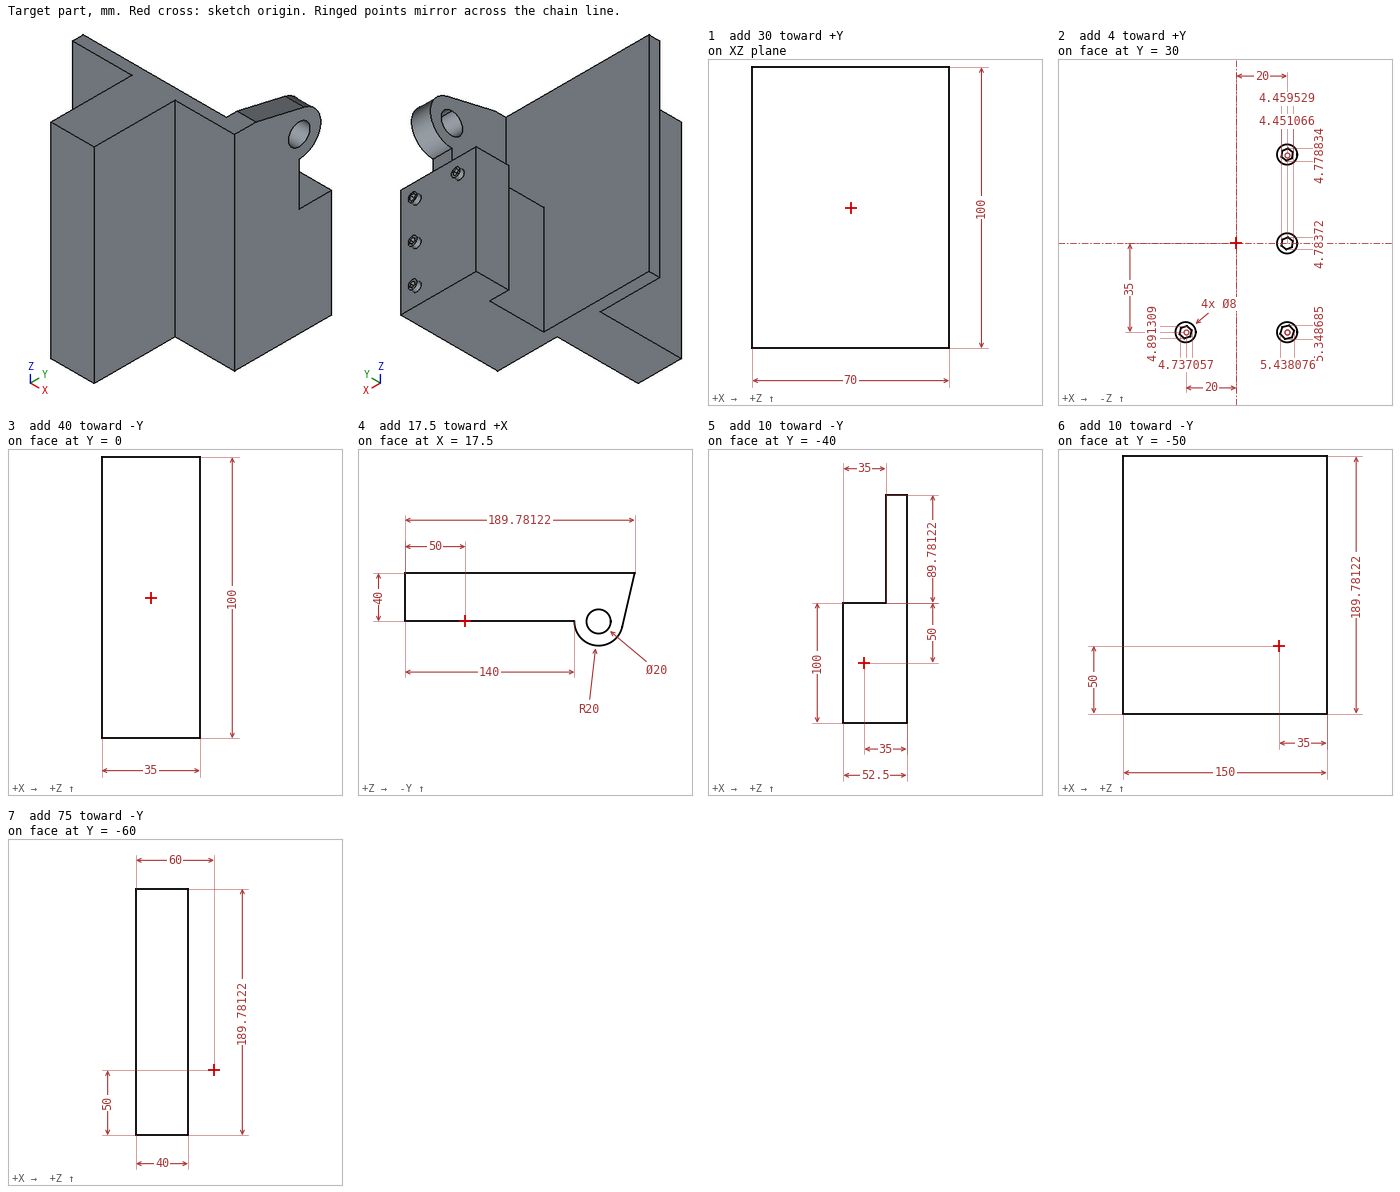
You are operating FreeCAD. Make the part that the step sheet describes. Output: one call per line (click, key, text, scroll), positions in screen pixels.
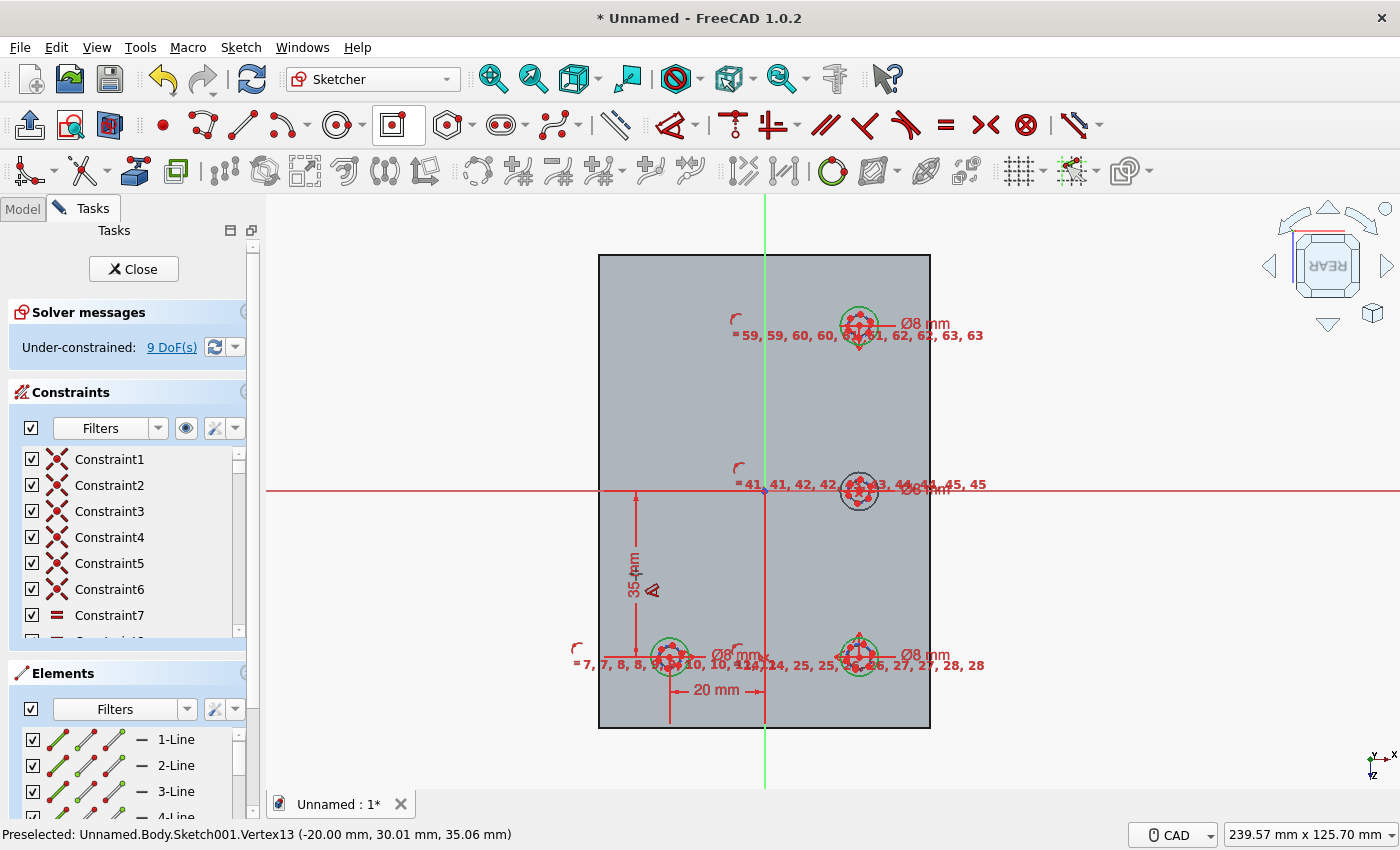
click(859, 491)
click(812, 525)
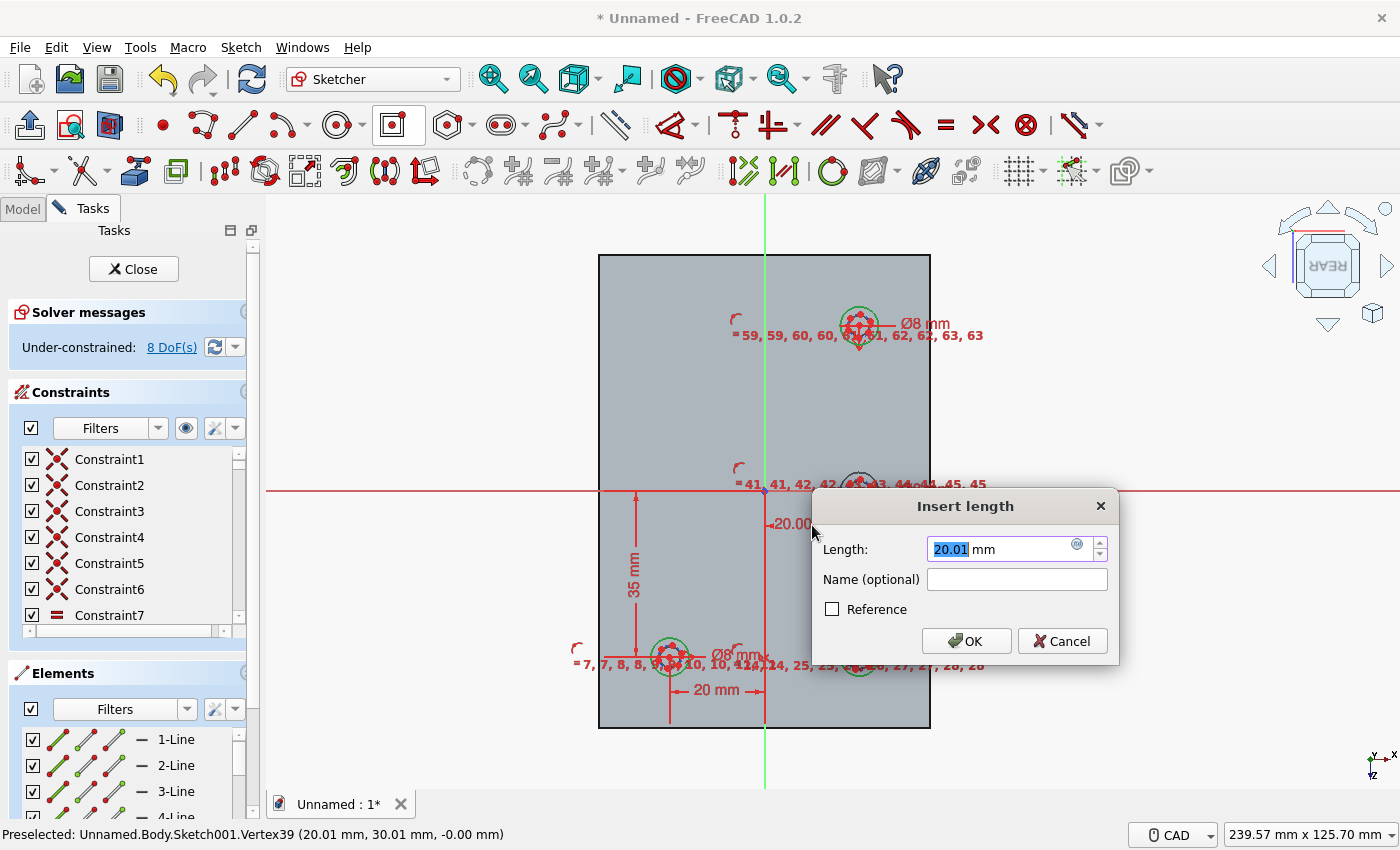
text(20)
key(Return)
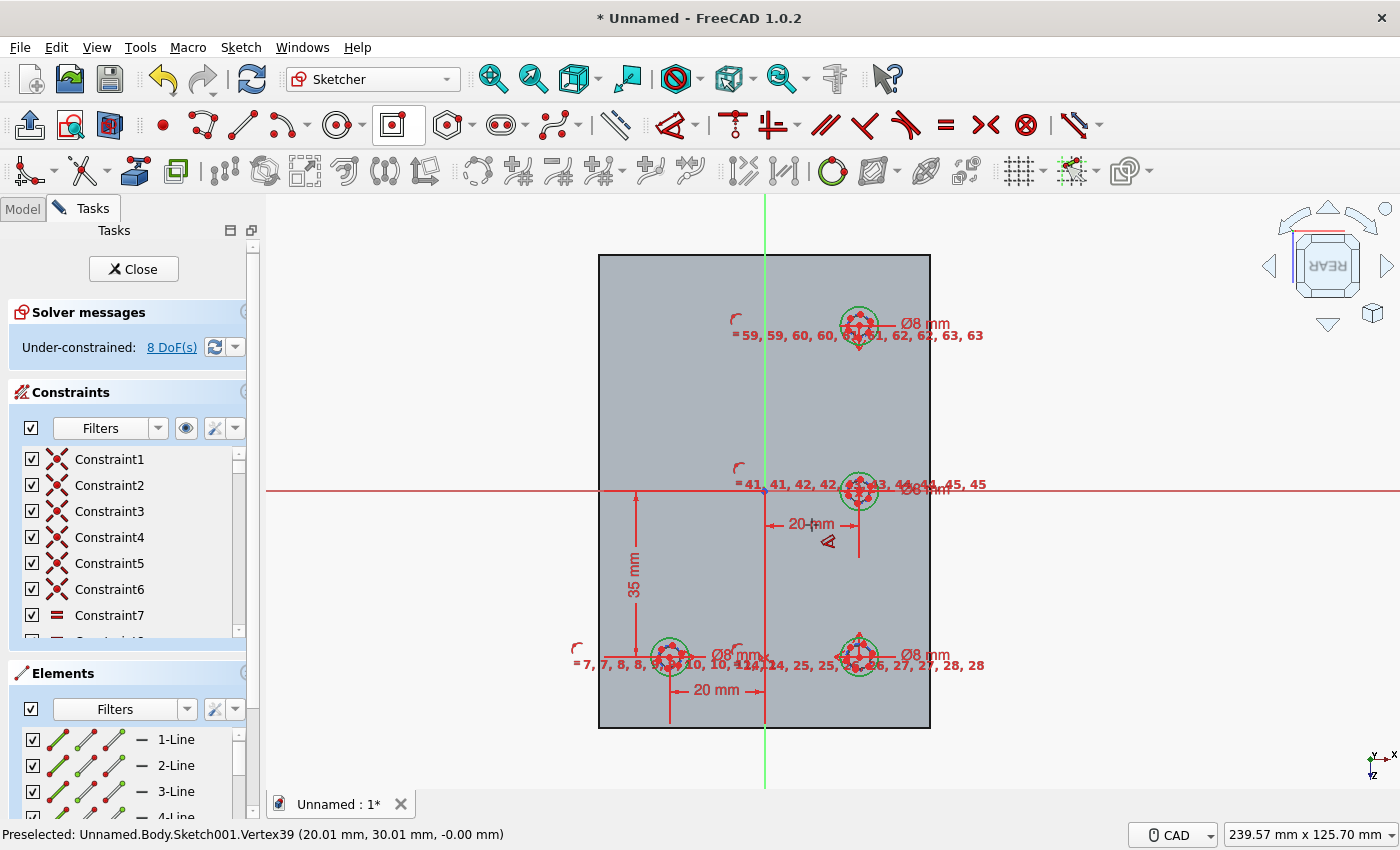
scroll(659, 660, up, 3)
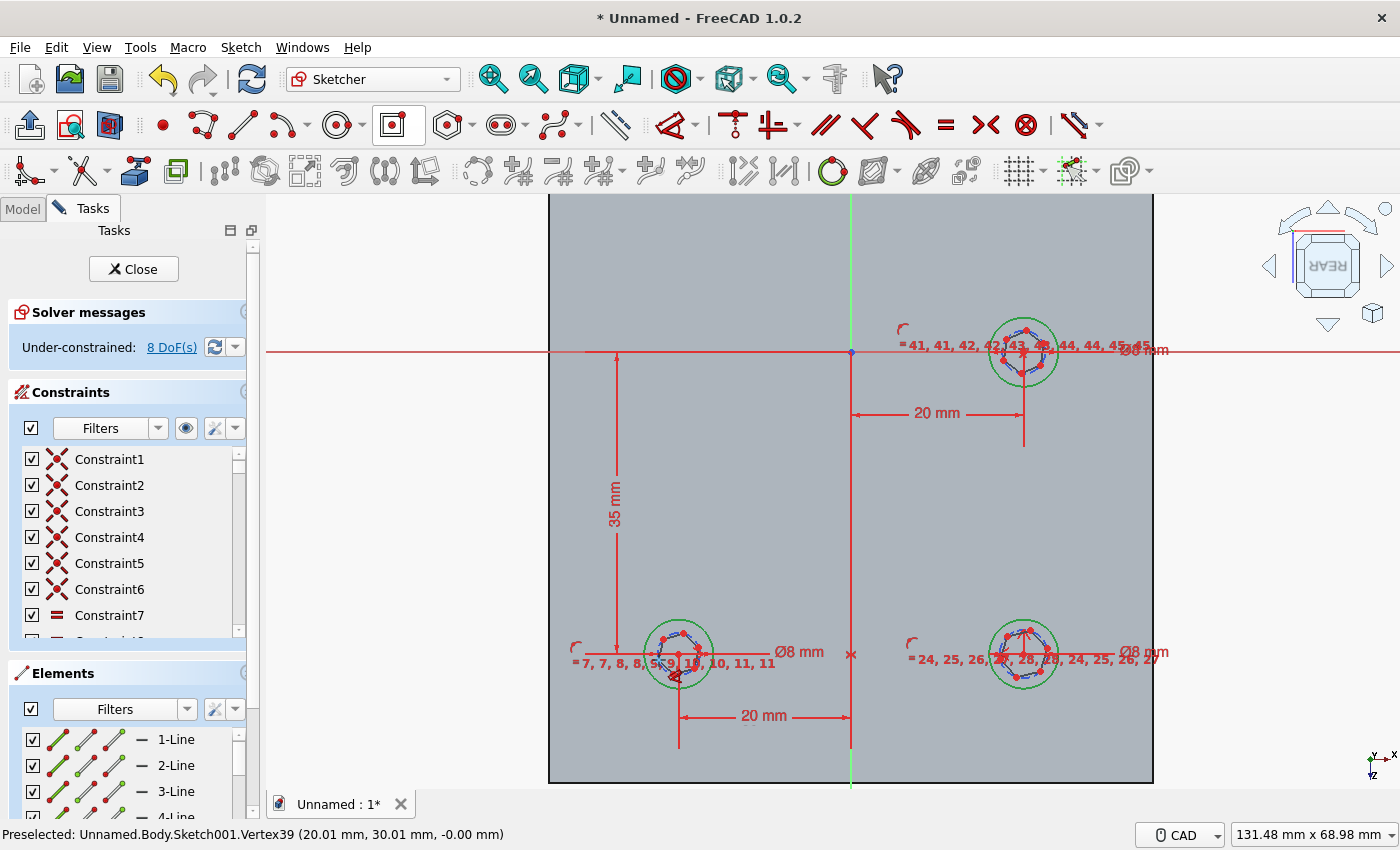
click(659, 660)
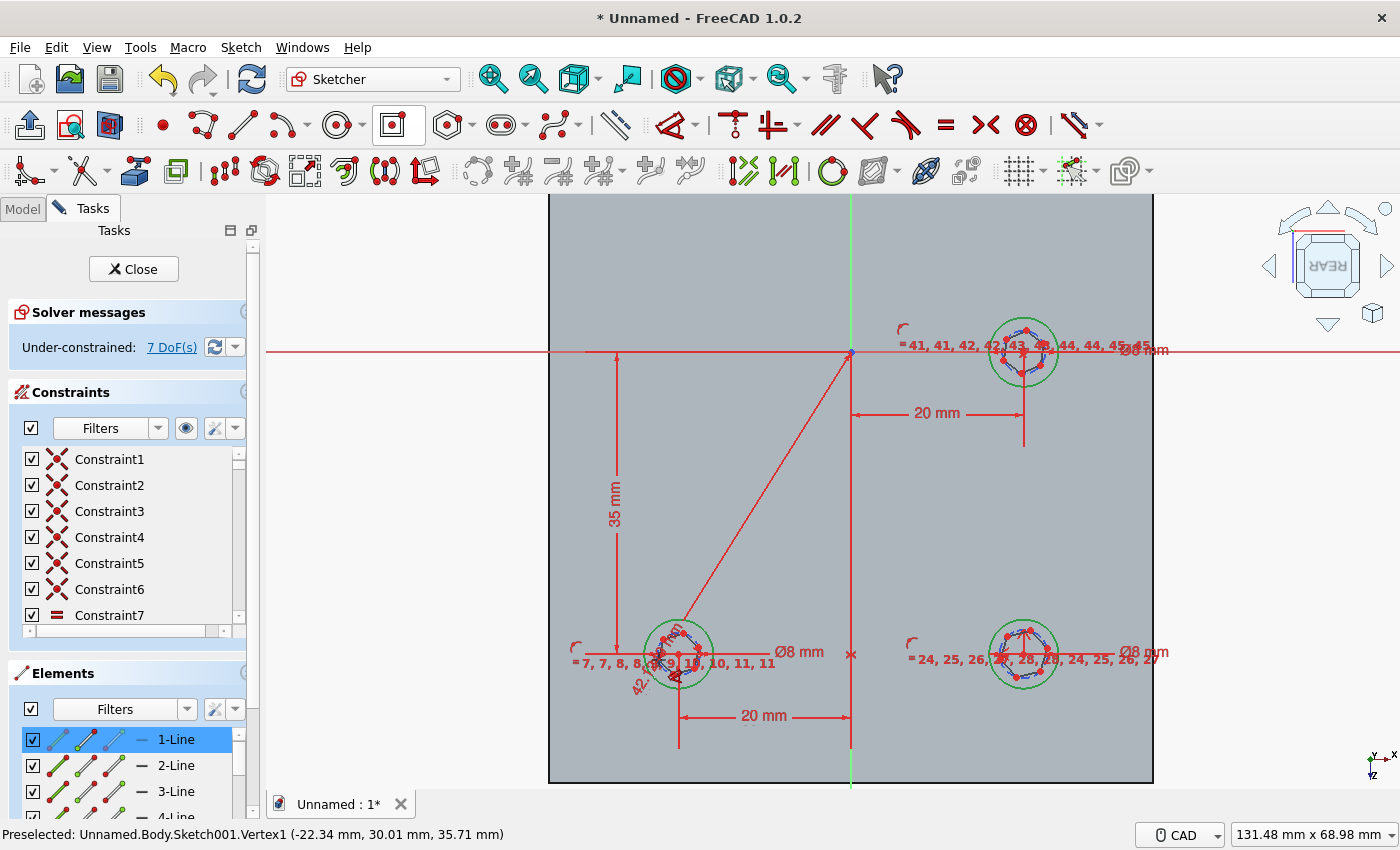
click(699, 648)
click(679, 718)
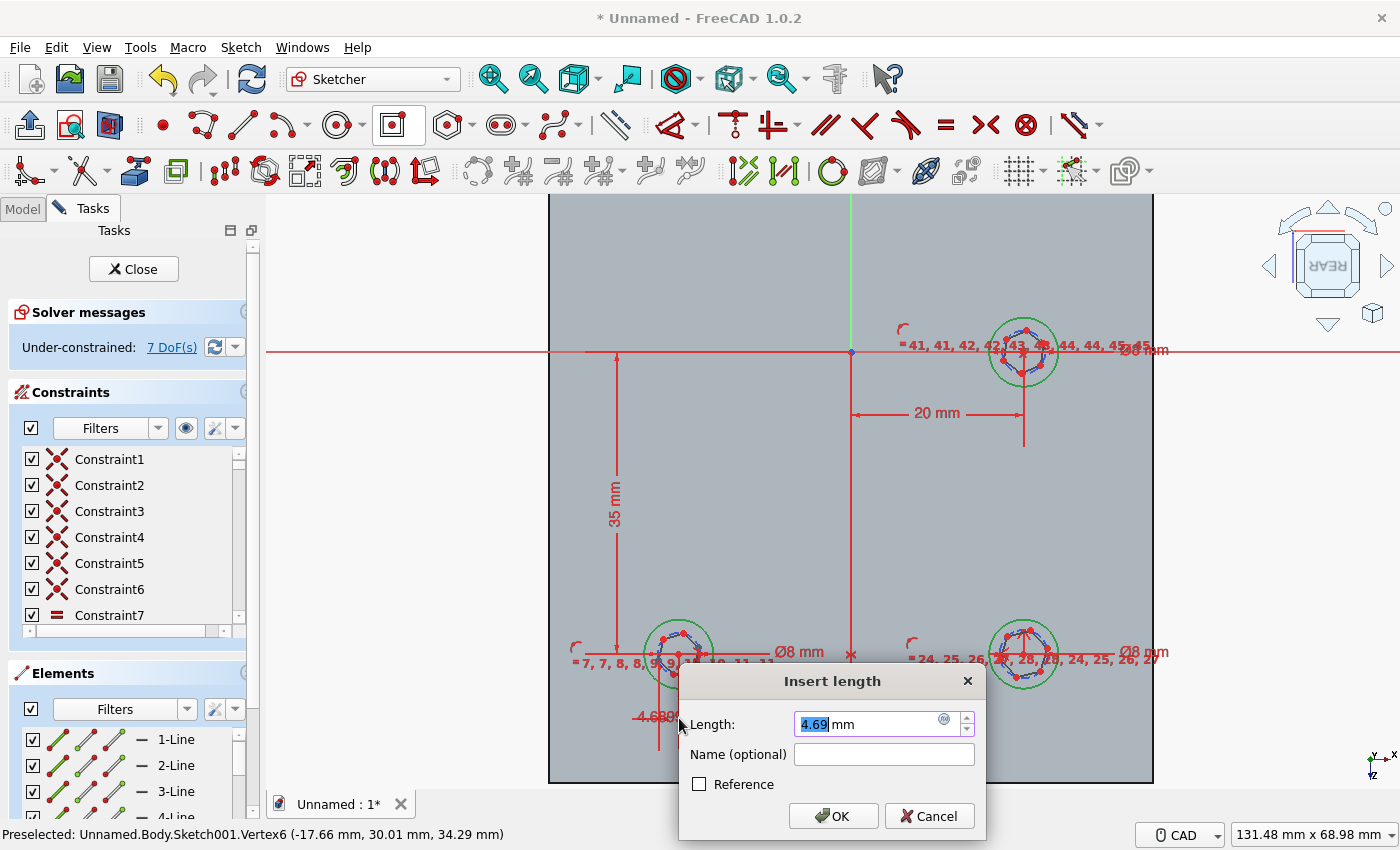
text(4.737057)
key(Return)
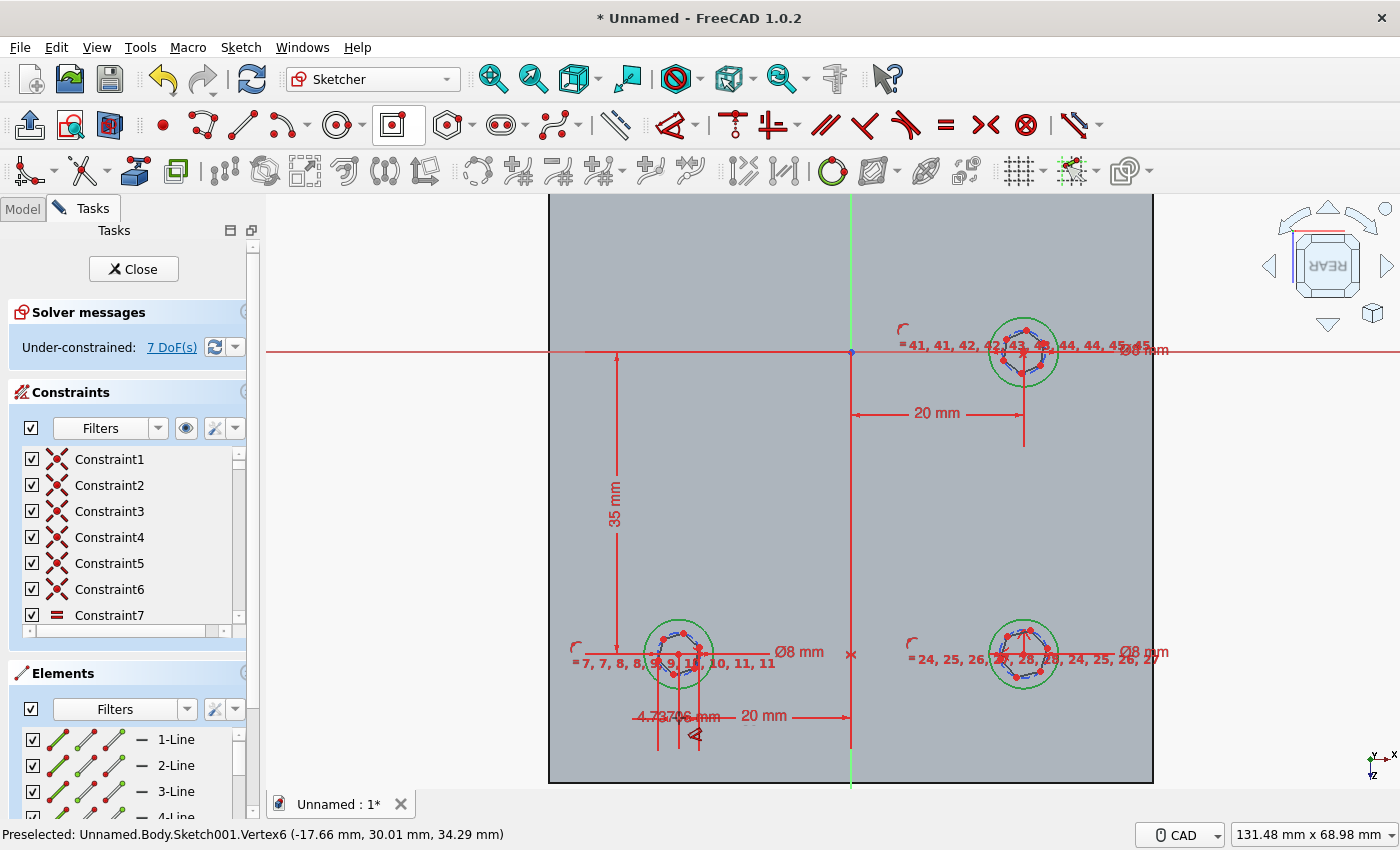
click(674, 675)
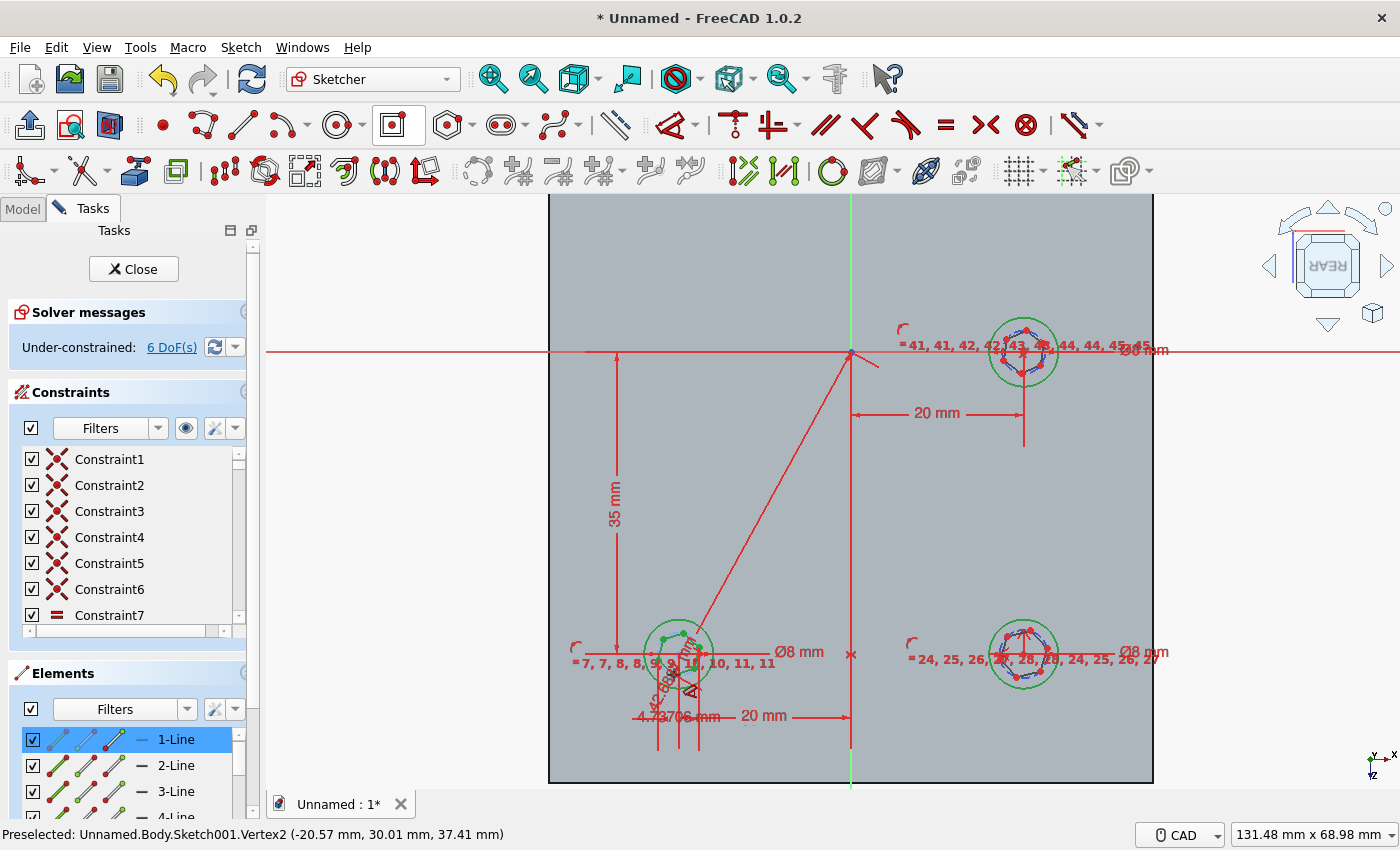
click(684, 633)
click(616, 654)